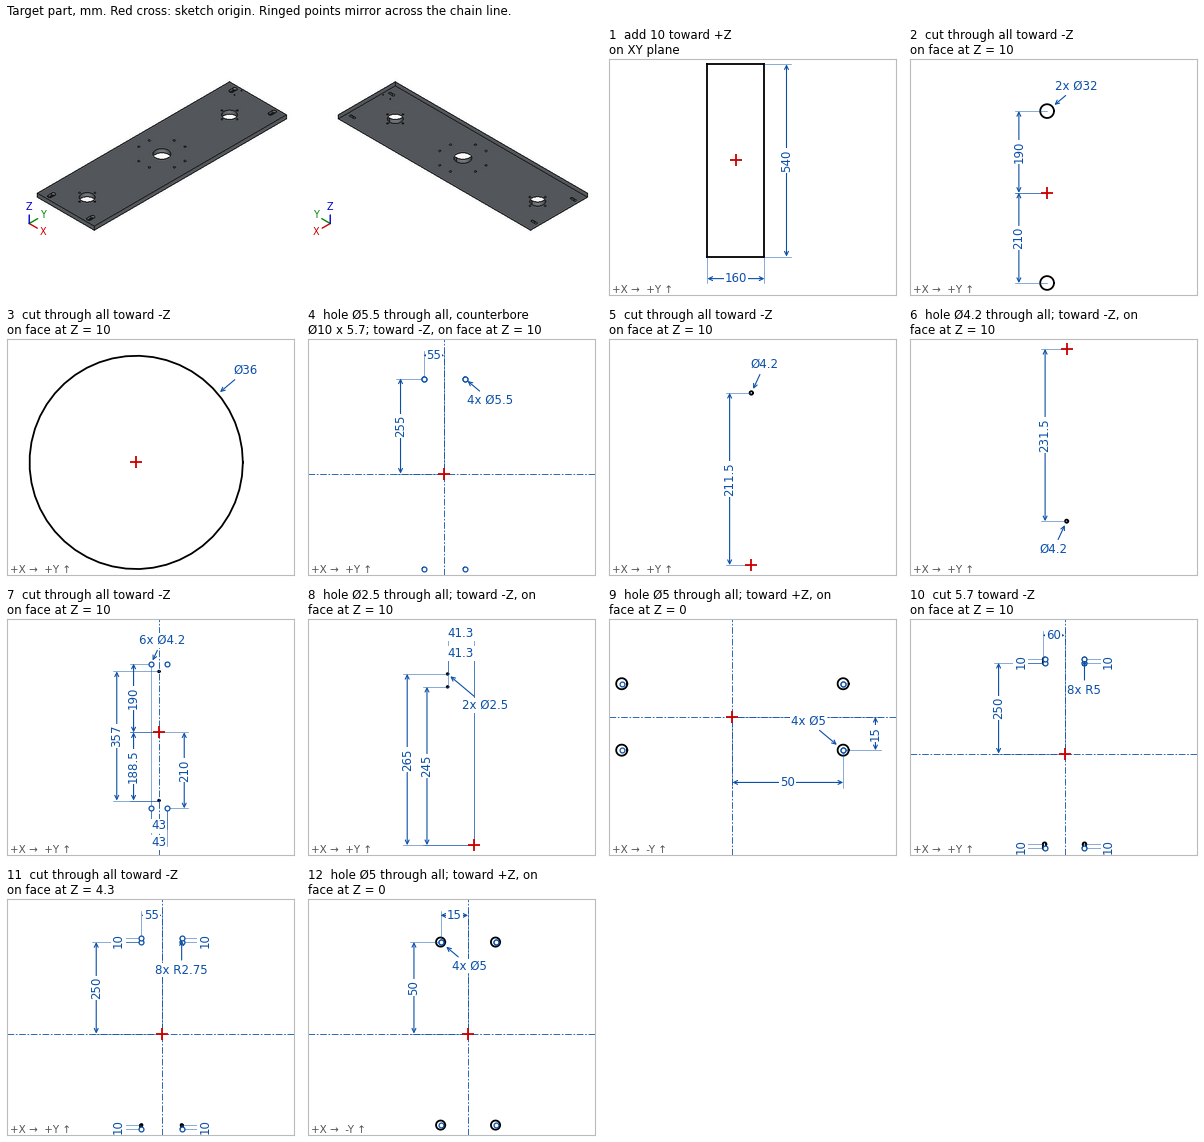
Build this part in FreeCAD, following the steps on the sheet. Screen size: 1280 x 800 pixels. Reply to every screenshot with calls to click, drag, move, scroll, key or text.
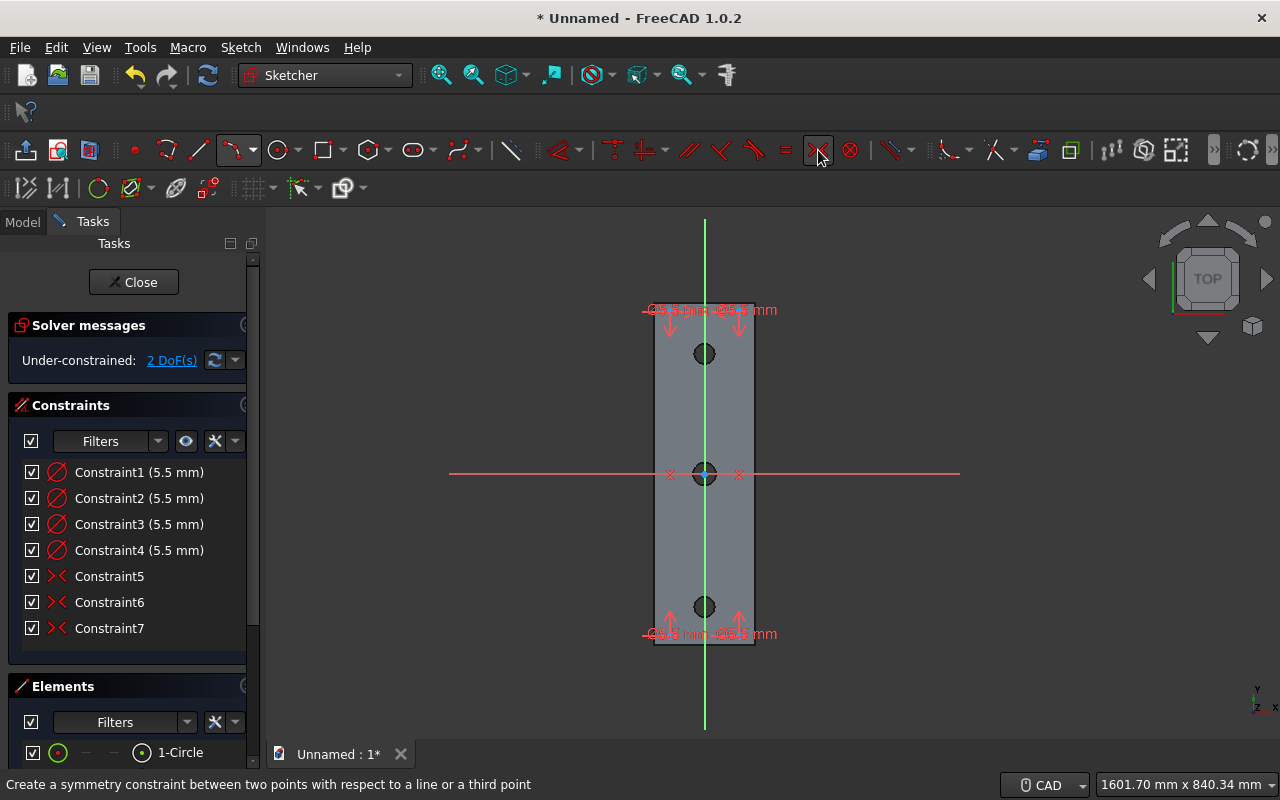
click(558, 150)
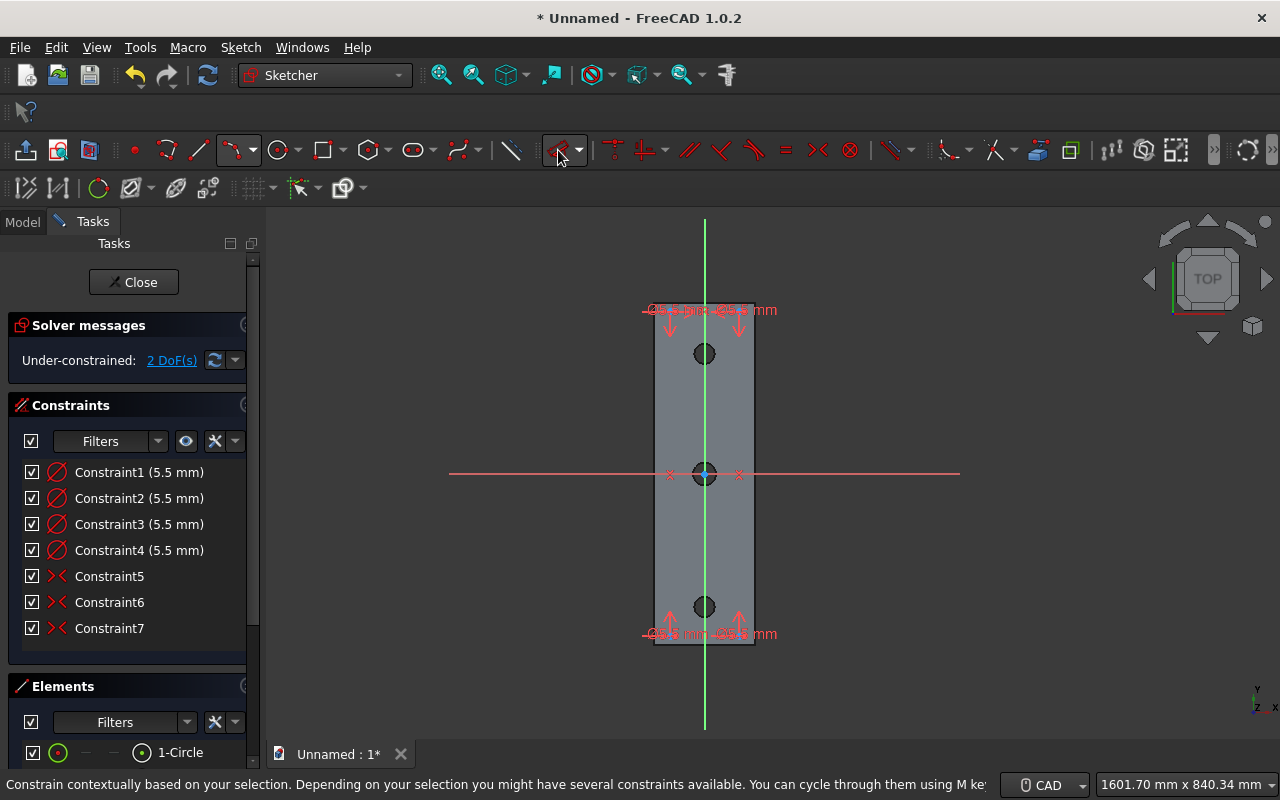
click(670, 312)
click(687, 278)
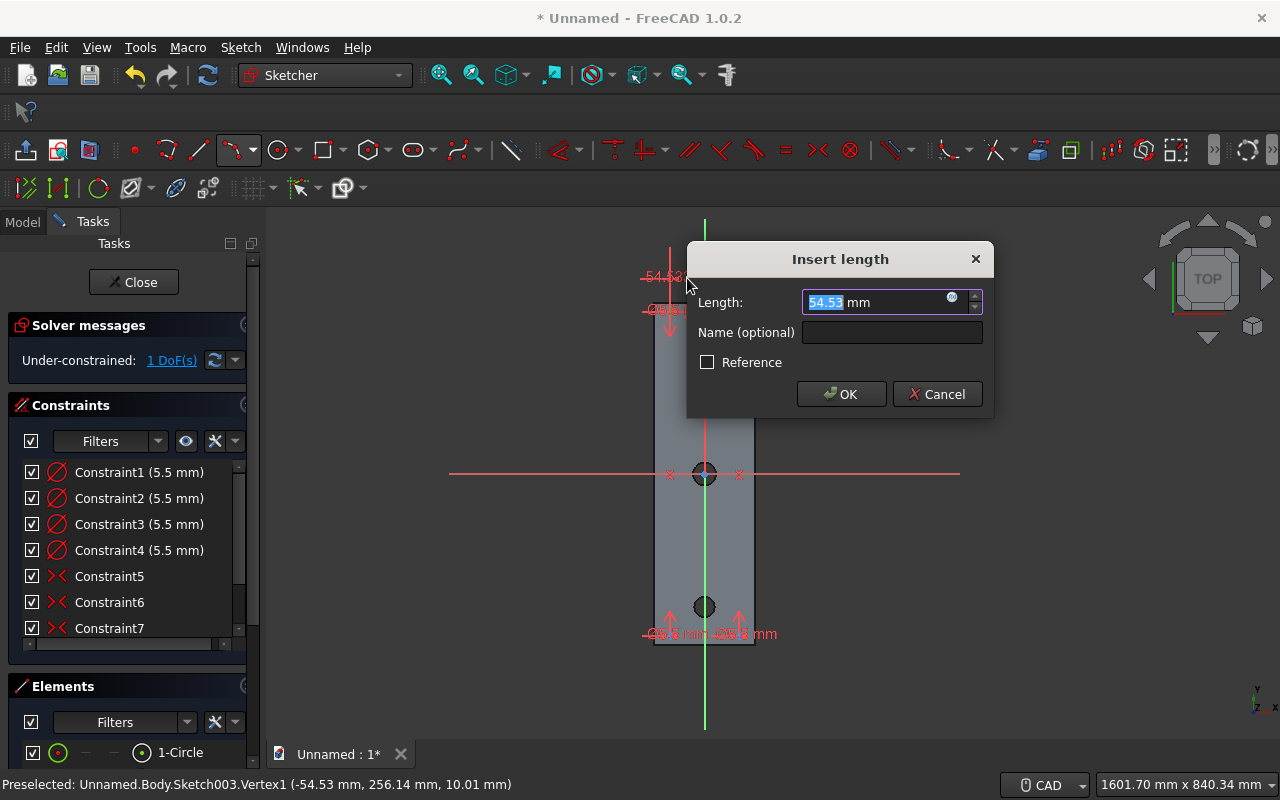
text(55)
key(Return)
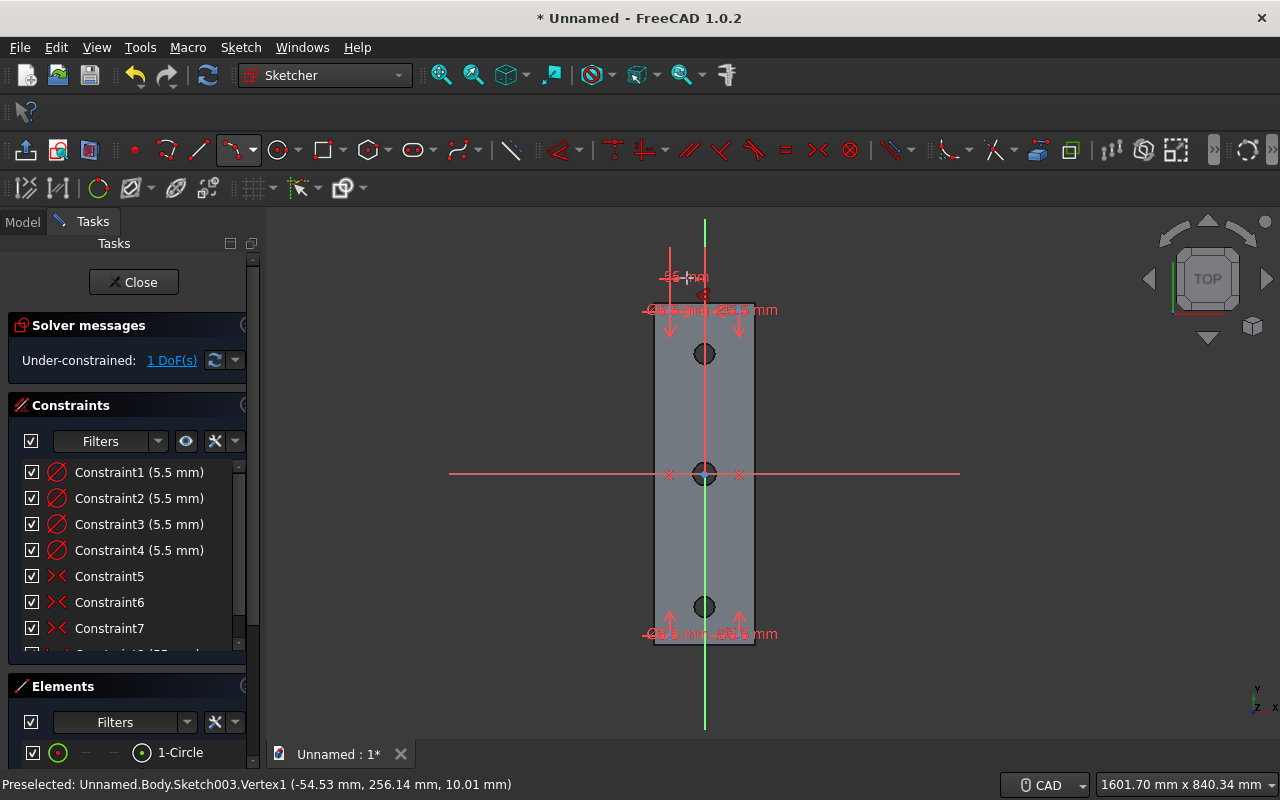
click(670, 312)
click(636, 393)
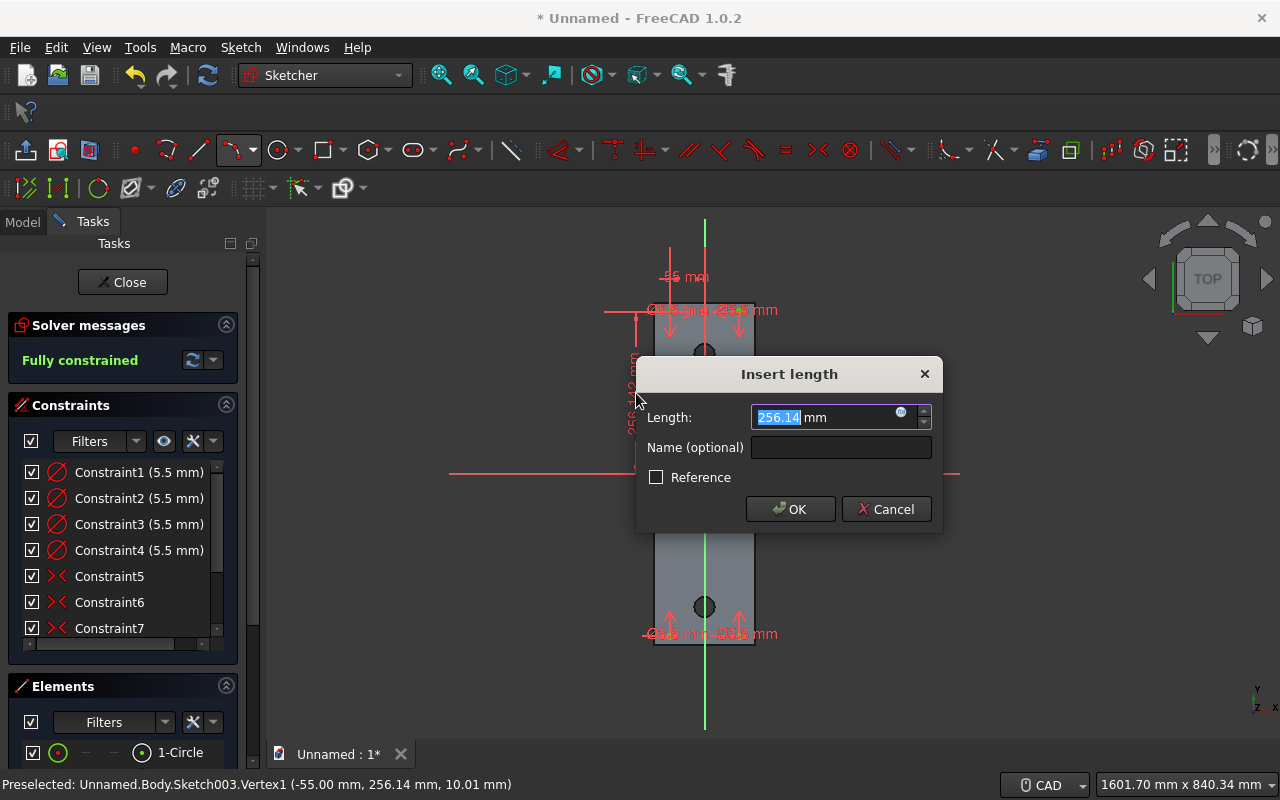
text(255)
key(Return)
key(Escape)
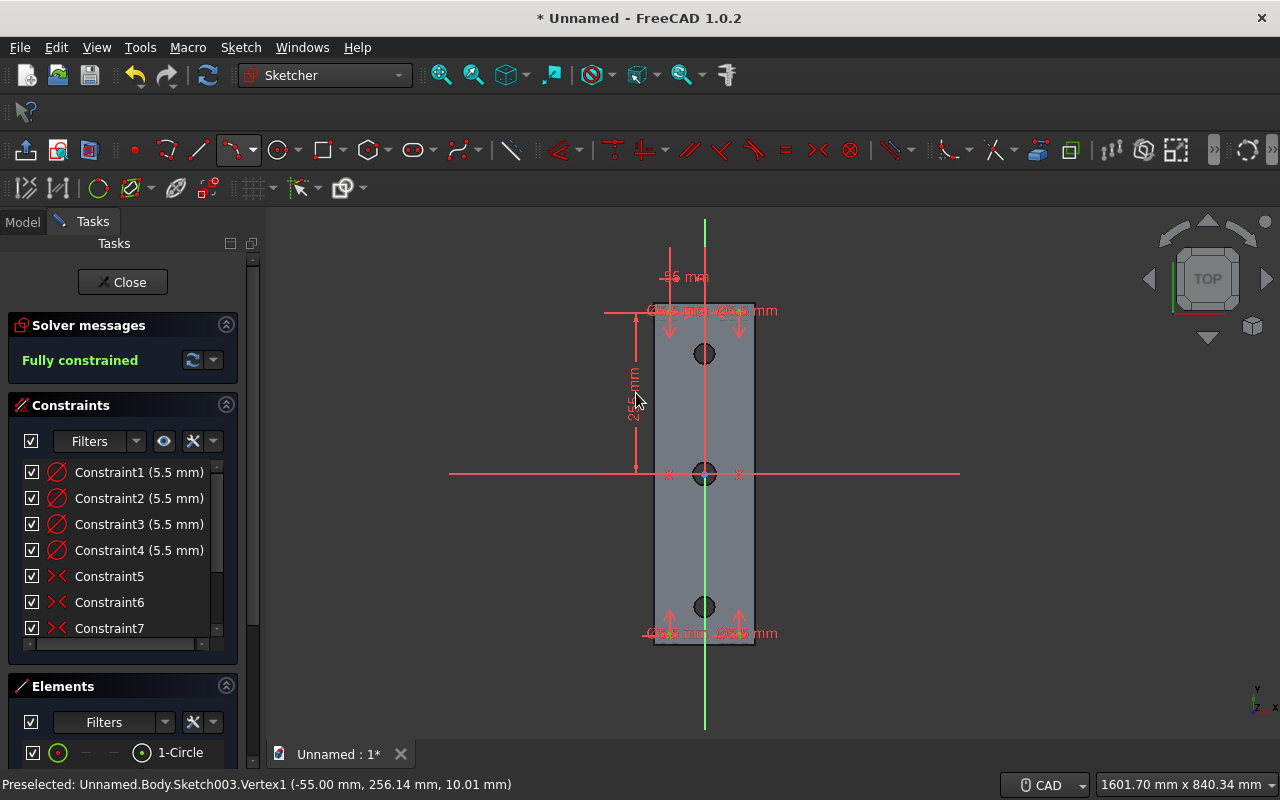
click(123, 282)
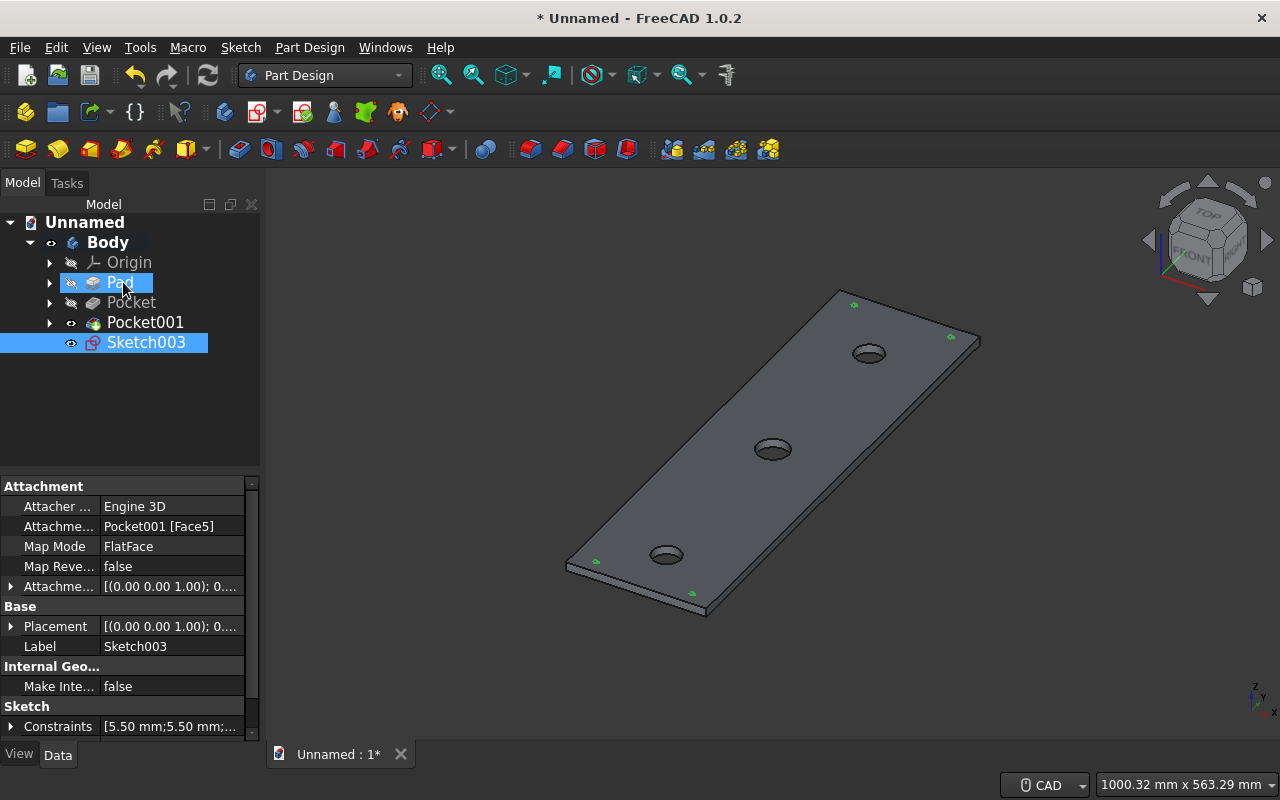
click(272, 150)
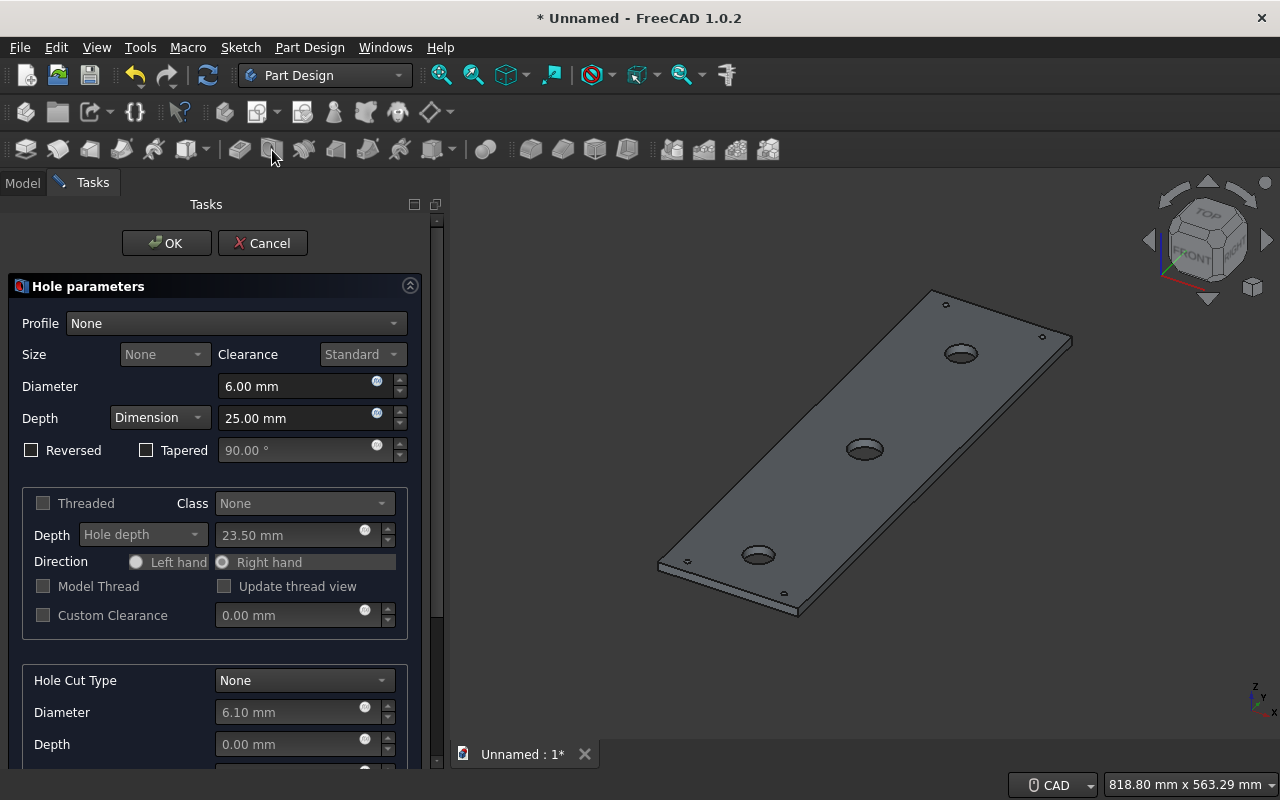
triple_click(305, 386)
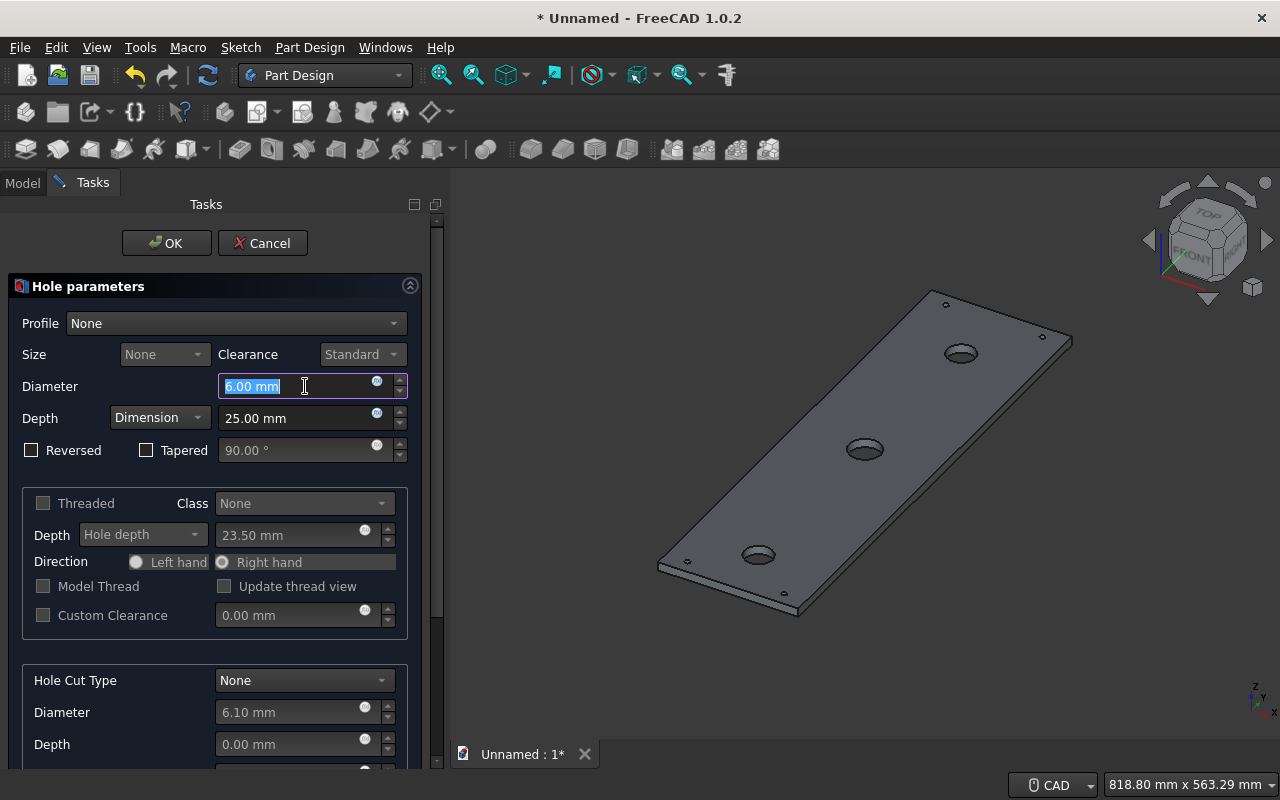
text(5.5)
key(Tab)